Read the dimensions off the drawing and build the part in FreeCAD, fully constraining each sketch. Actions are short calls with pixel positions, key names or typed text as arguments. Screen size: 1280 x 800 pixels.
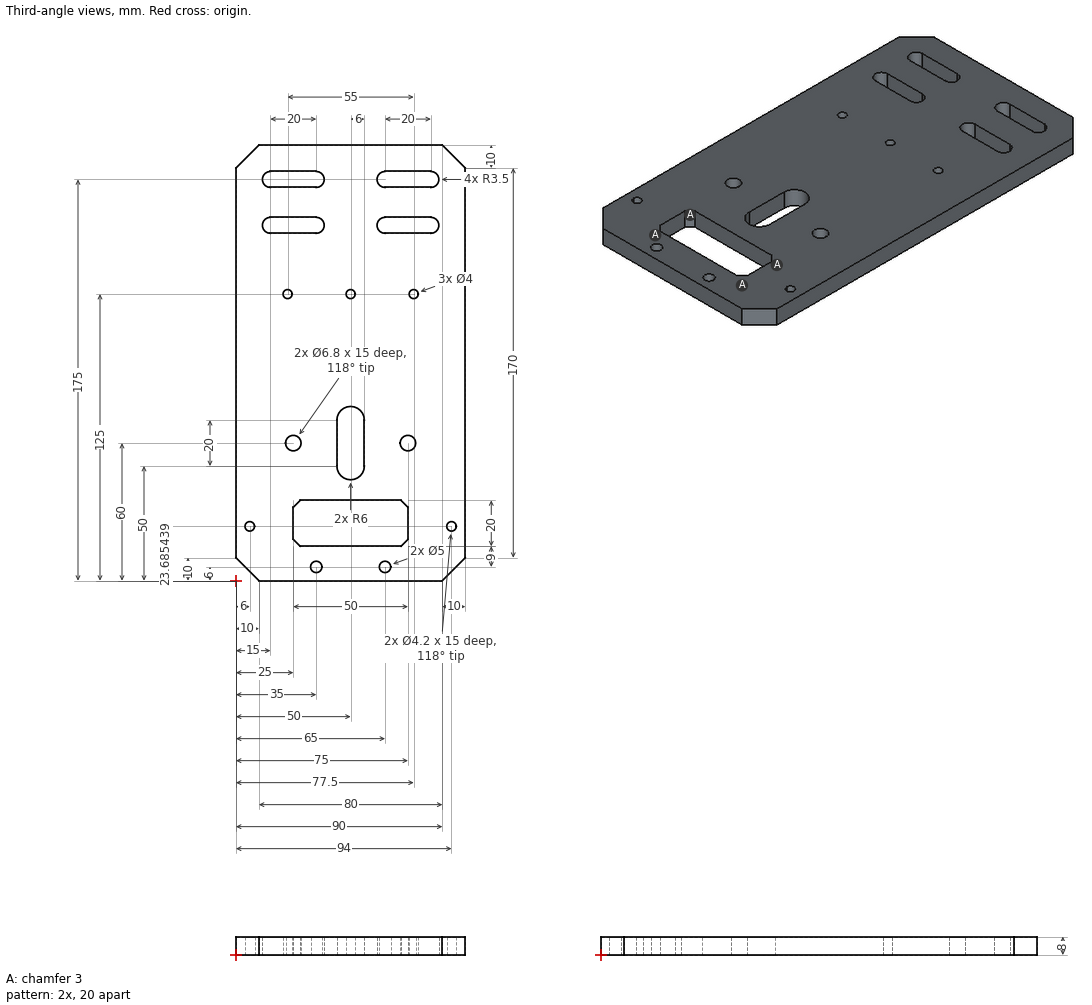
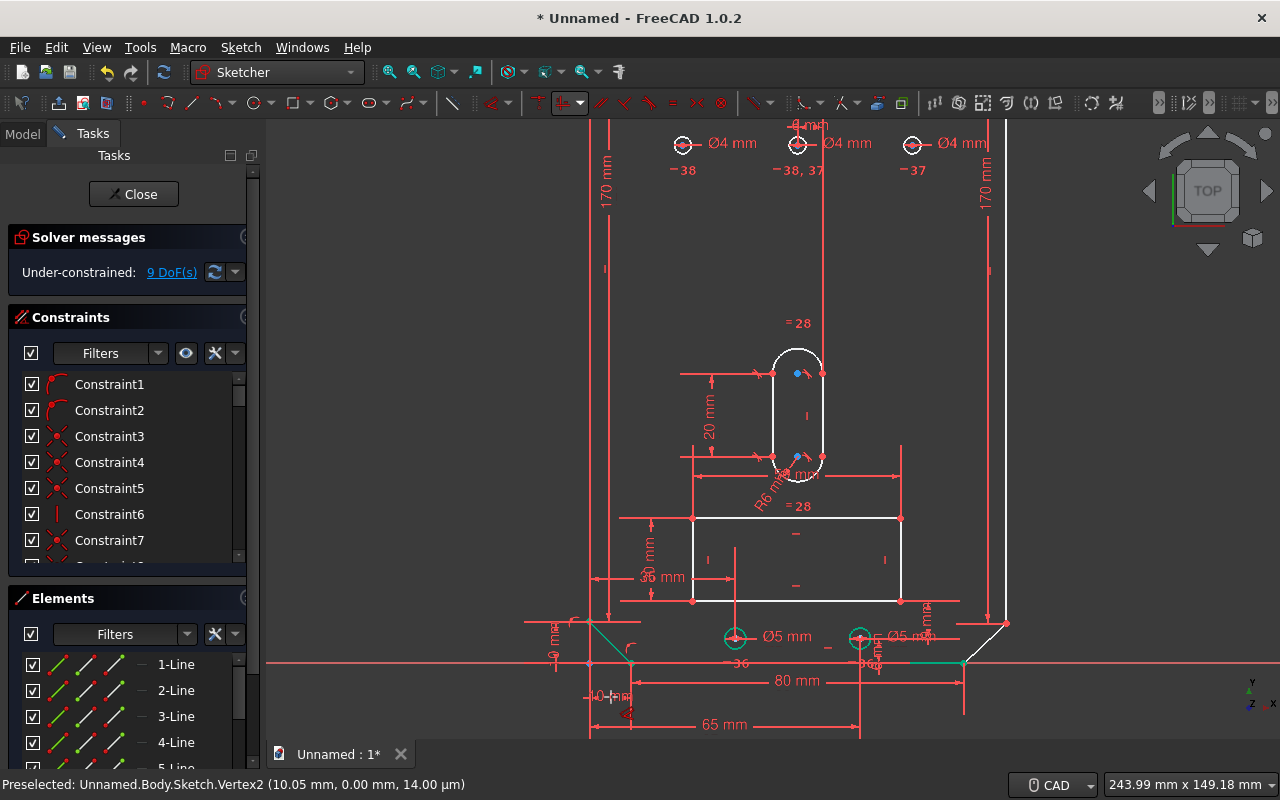
click(1006, 624)
click(1040, 644)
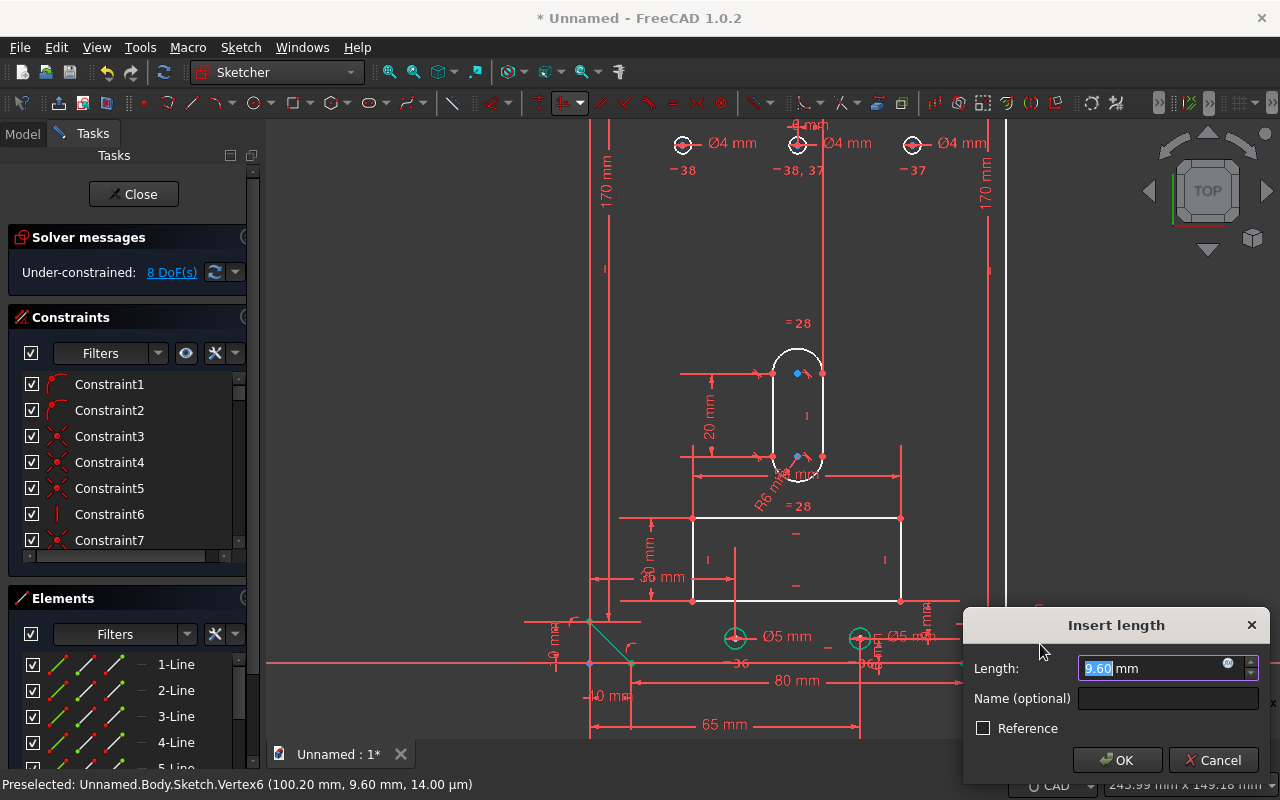
text(10)
key(Return)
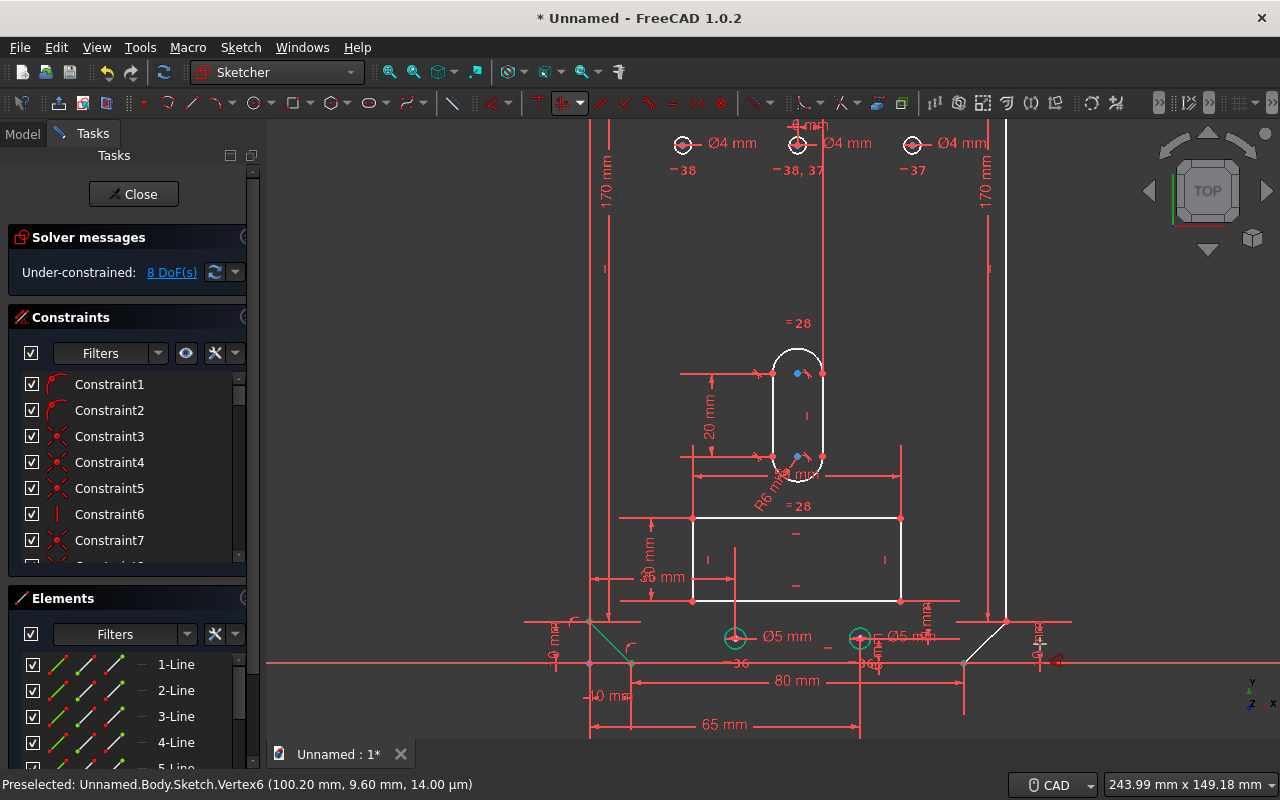
scroll(591, 624, down, 3)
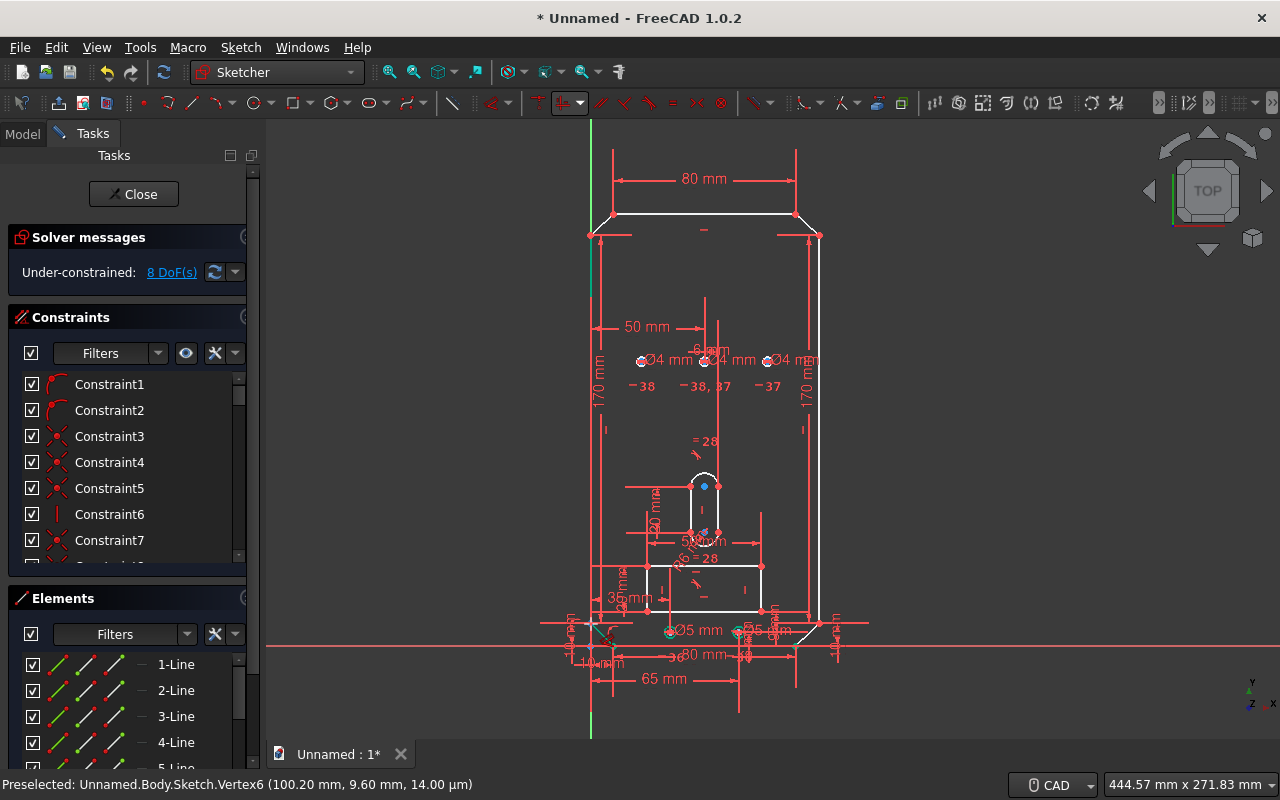
click(796, 214)
click(740, 680)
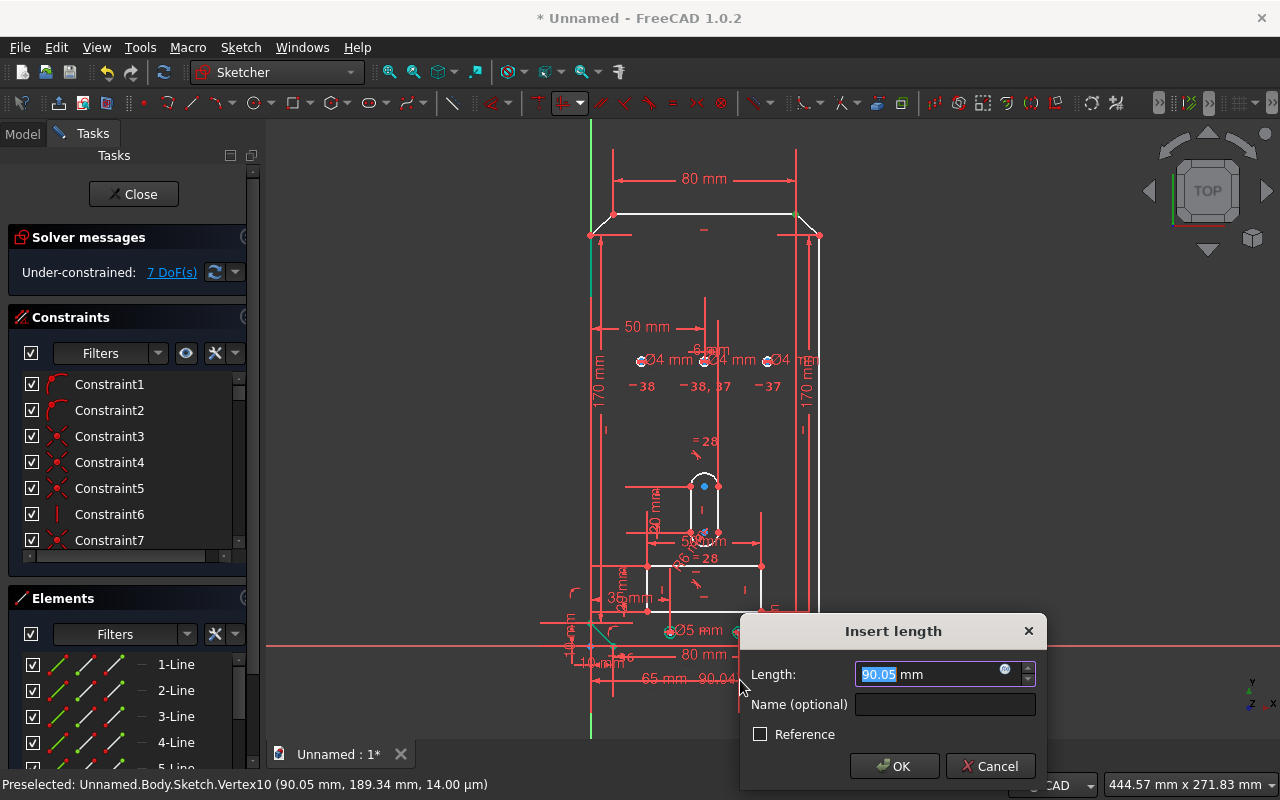
text(90)
key(Return)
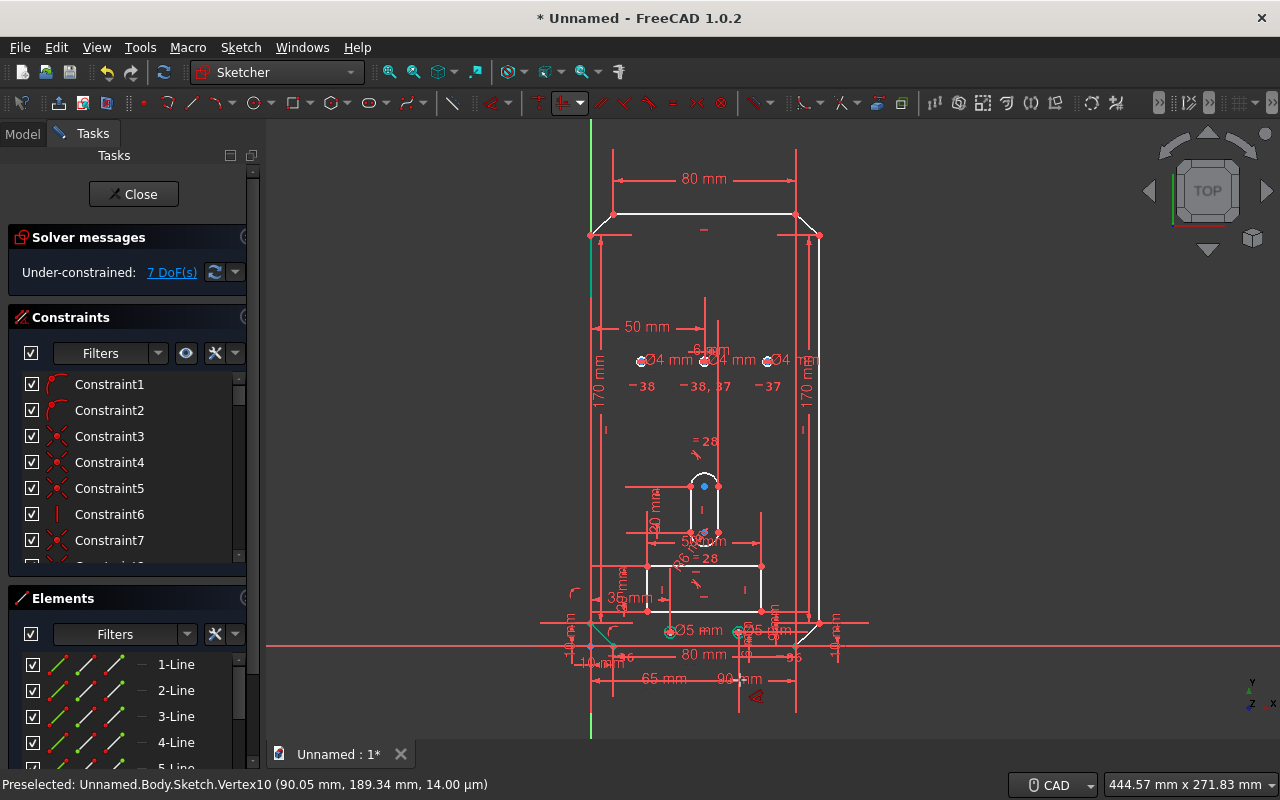
click(647, 566)
click(619, 532)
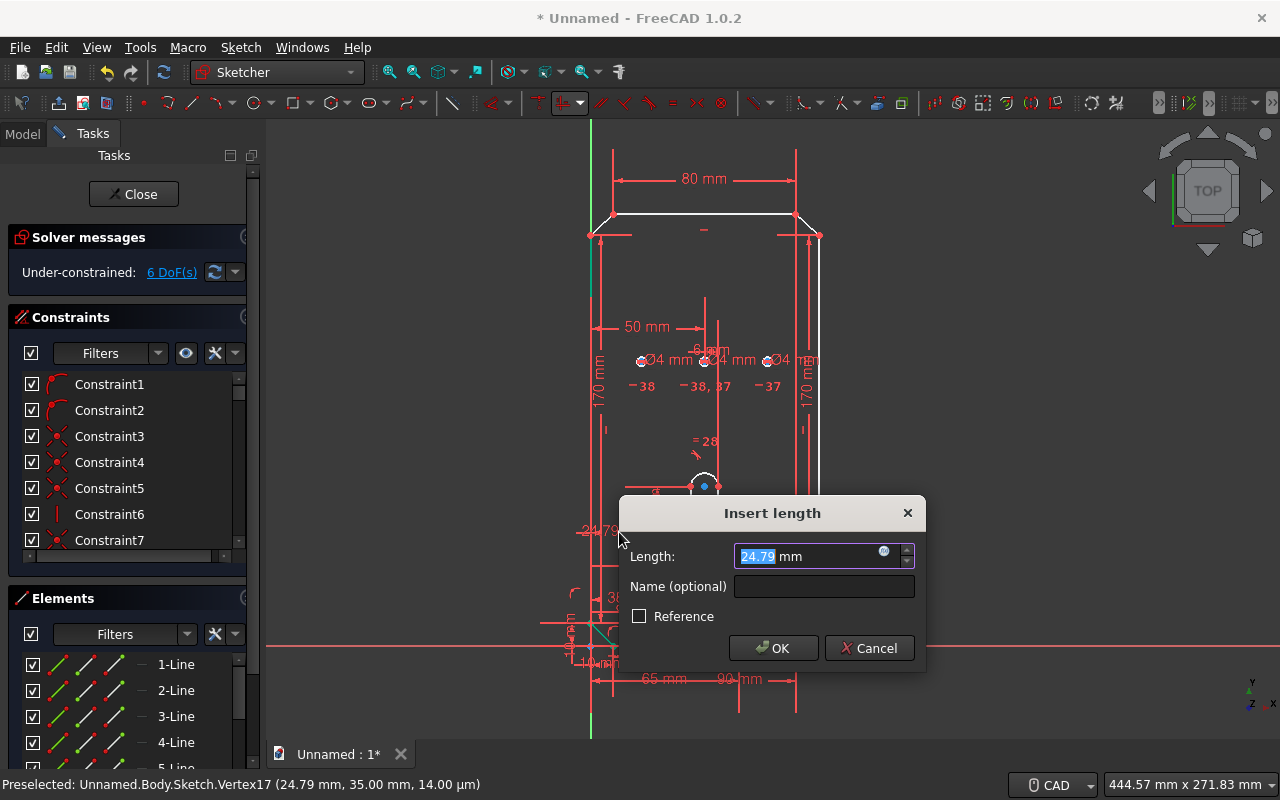
text(25)
key(Return)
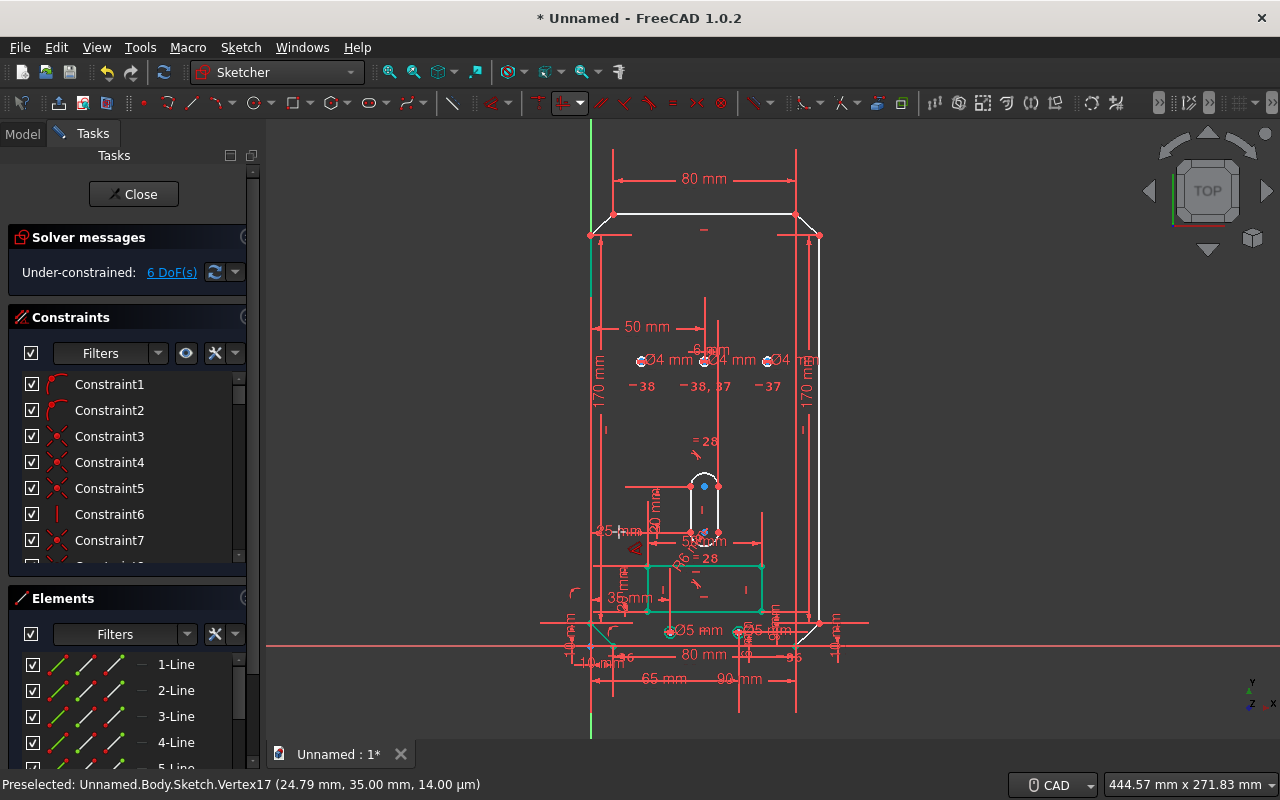
click(691, 533)
click(557, 589)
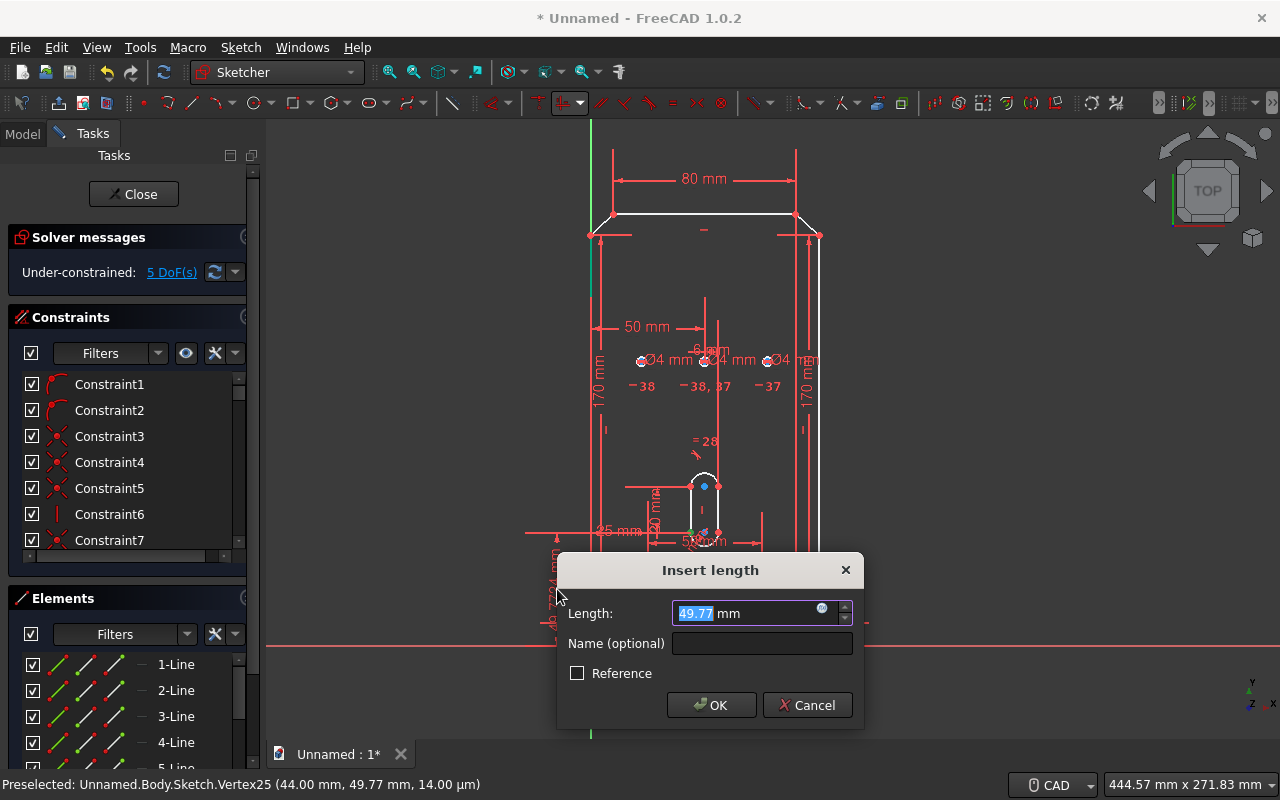
text(50)
key(Return)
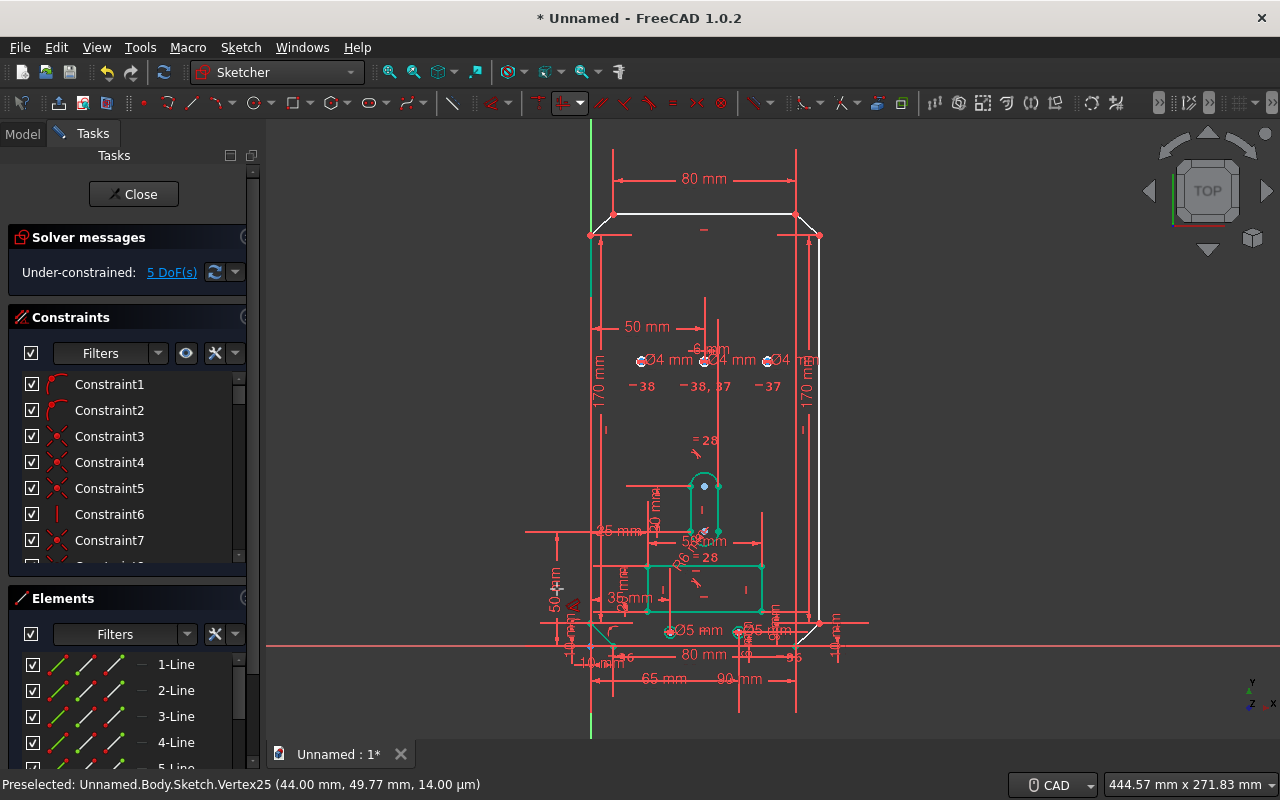
scroll(812, 630, up, 3)